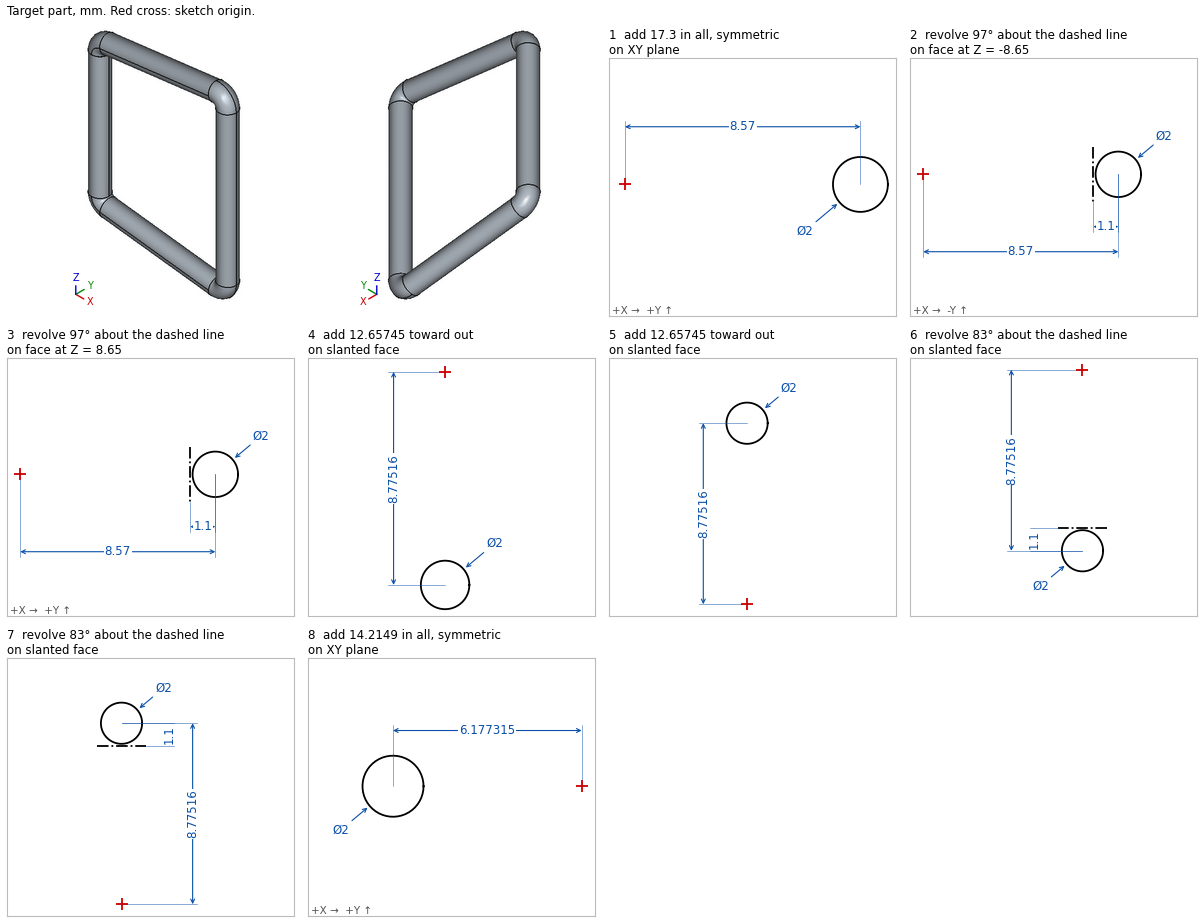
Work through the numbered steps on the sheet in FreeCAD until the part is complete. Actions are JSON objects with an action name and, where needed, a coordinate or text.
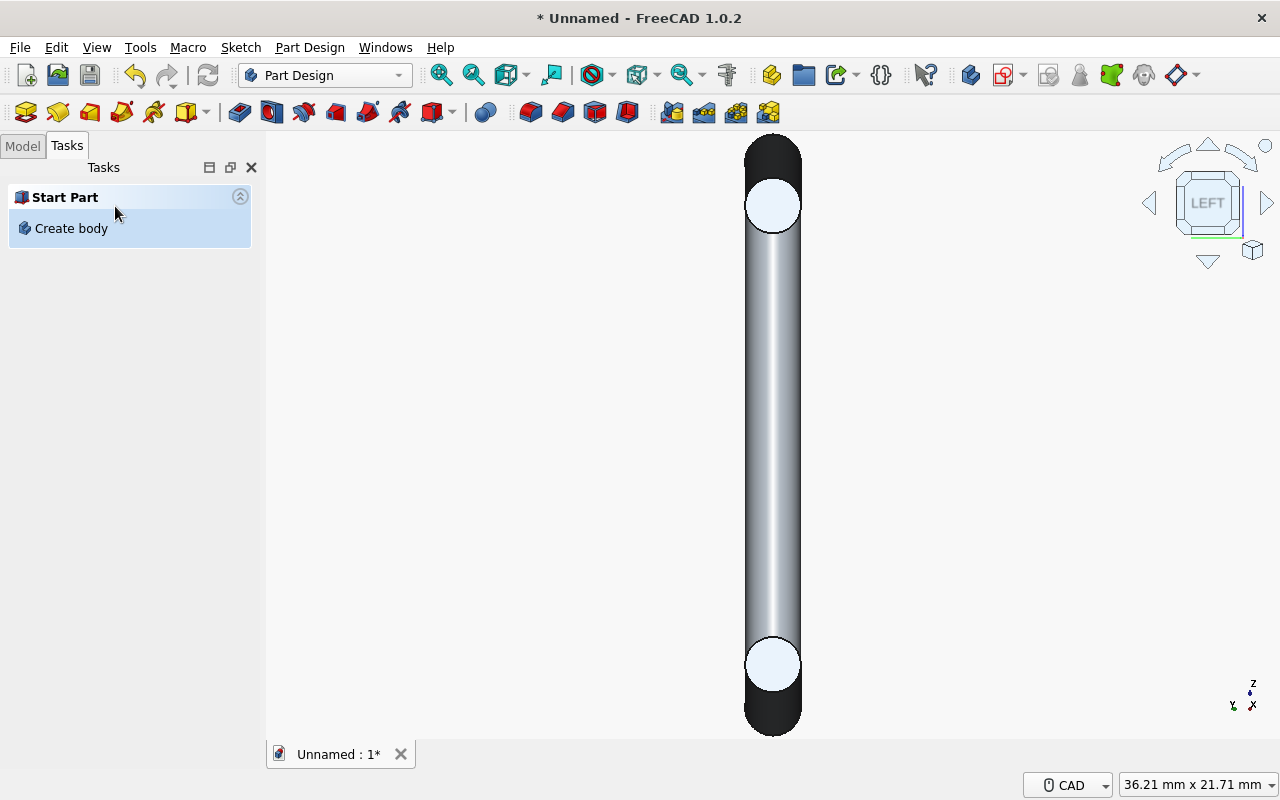
{"action": "left_click", "coordinate": [773, 664]}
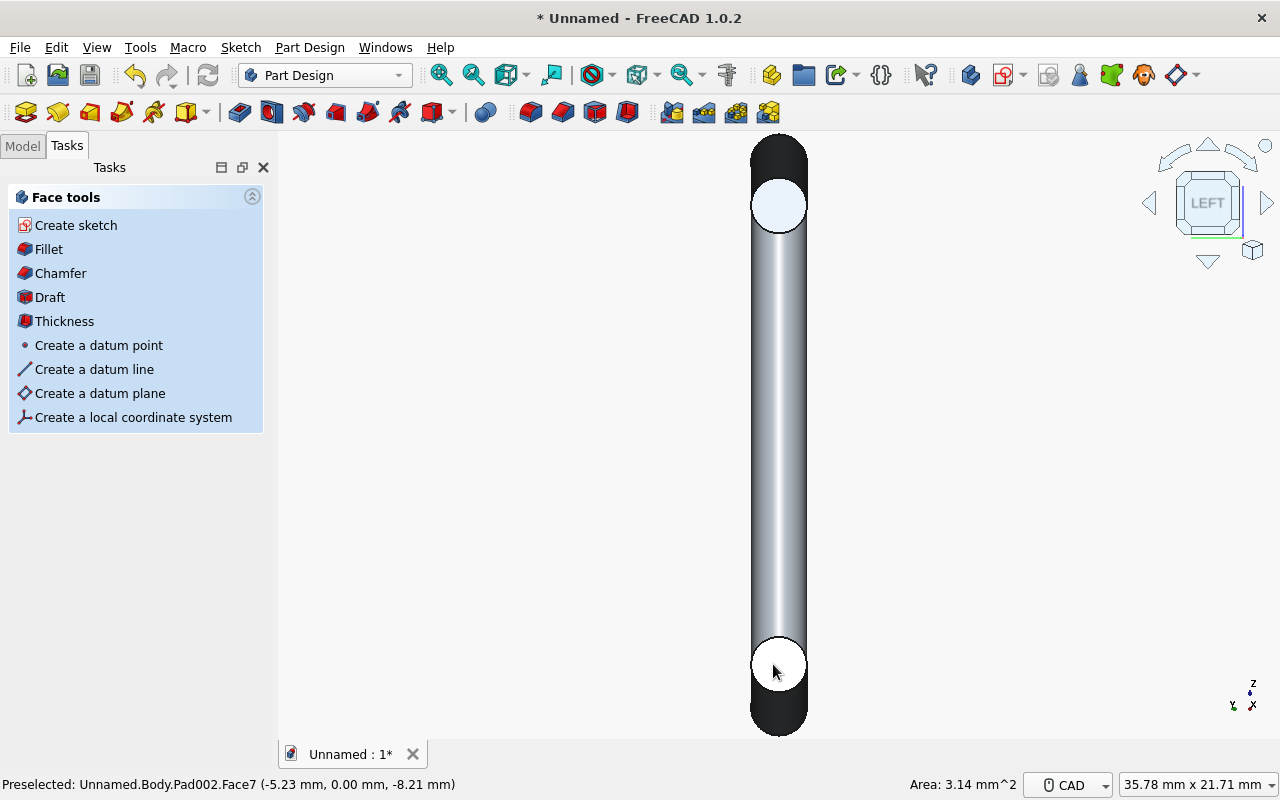
{"action": "left_click", "coordinate": [1004, 76]}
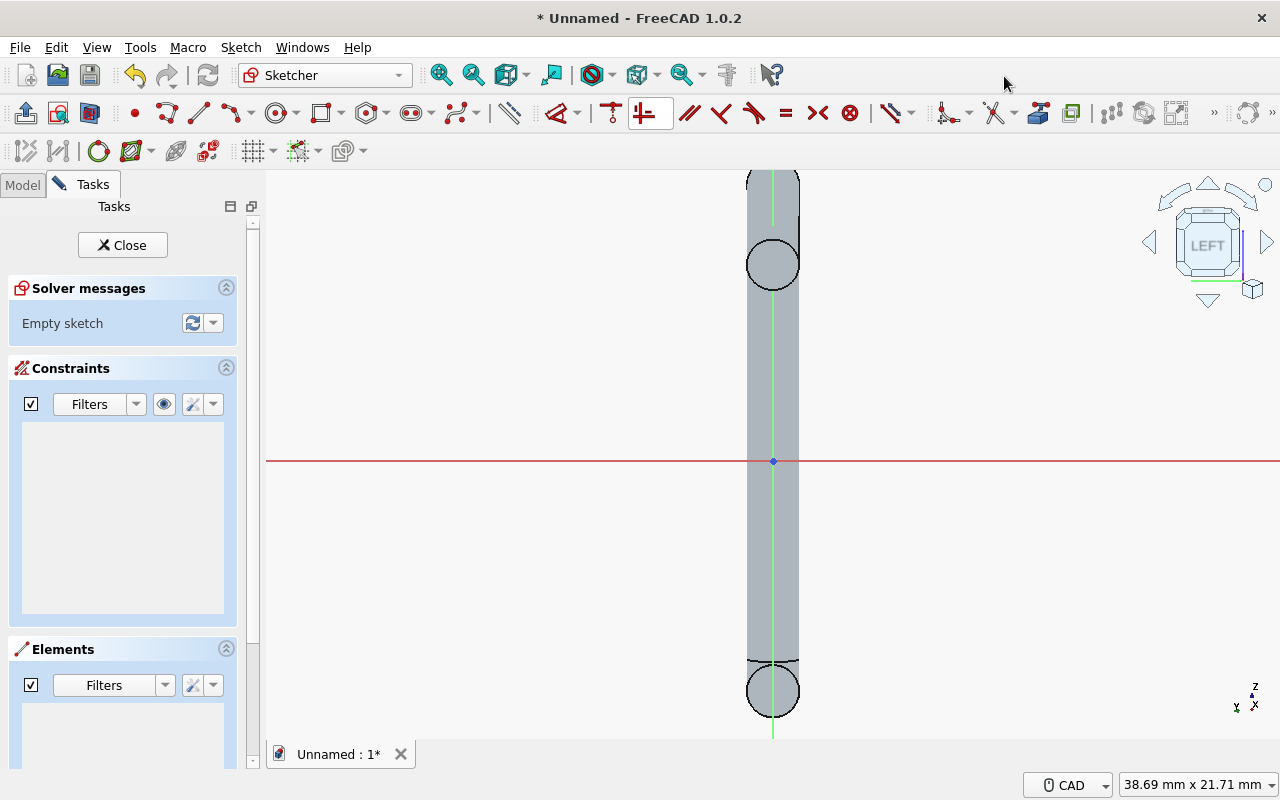
{"action": "scroll", "coordinate": [704, 454], "scroll_direction": "down", "scroll_amount": 5}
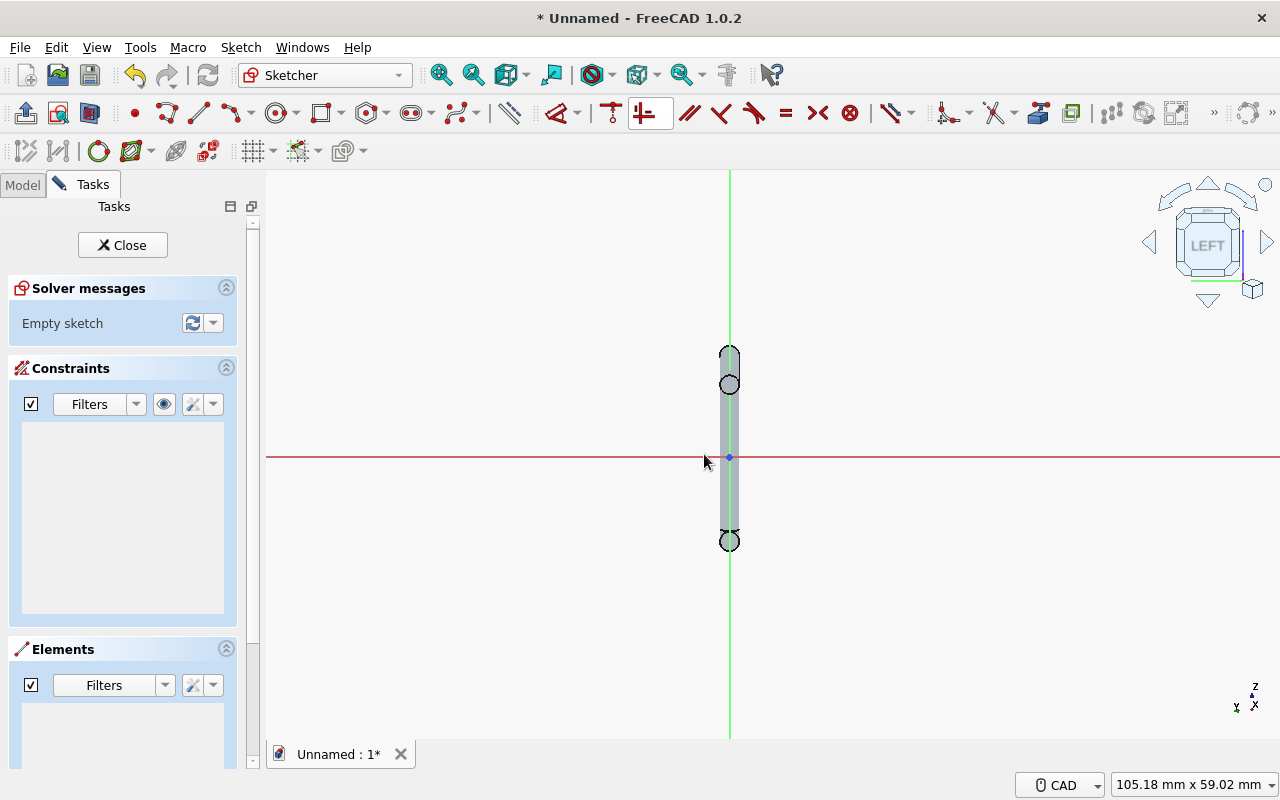
{"action": "scroll", "coordinate": [731, 547], "scroll_direction": "up", "scroll_amount": 14}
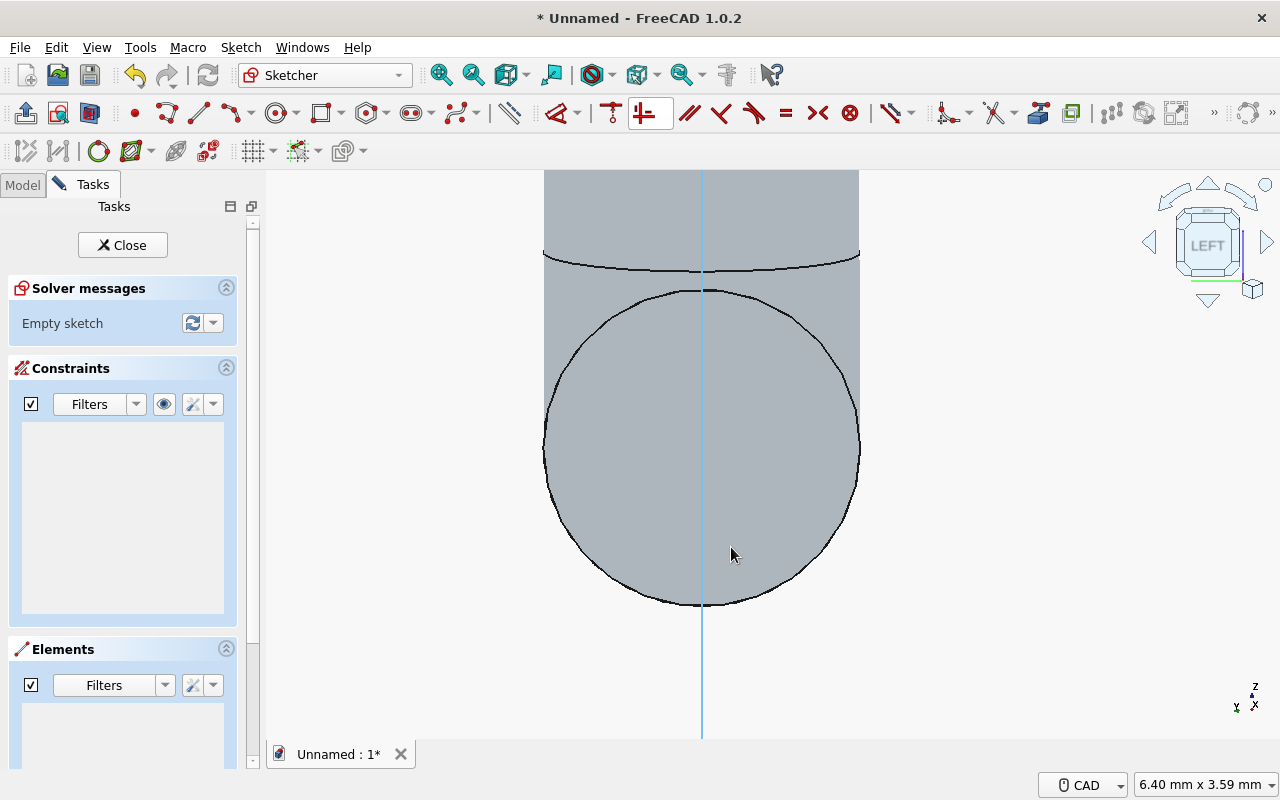
{"action": "left_click", "coordinate": [276, 114]}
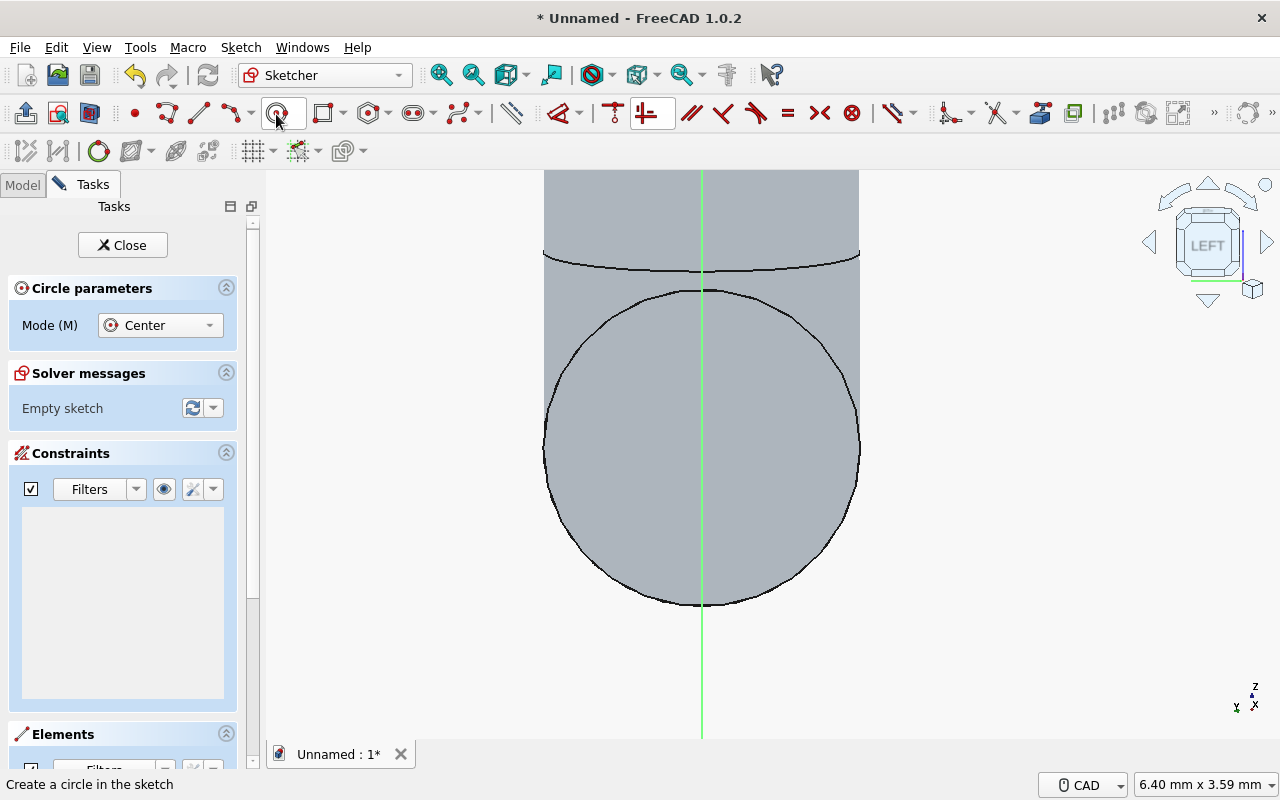
{"action": "left_click", "coordinate": [702, 448]}
{"action": "mouse_move", "coordinate": [814, 336]}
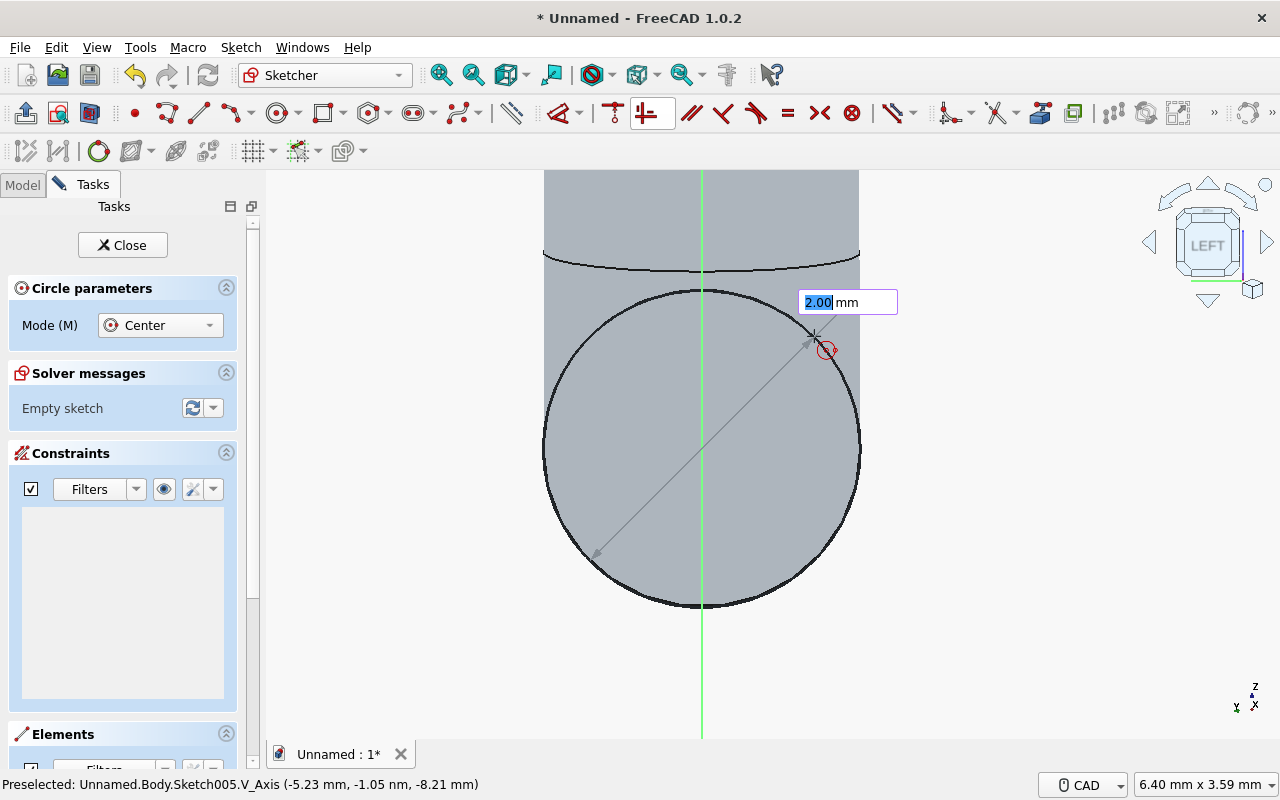
{"action": "type", "text": "2"}
{"action": "key", "text": "Return"}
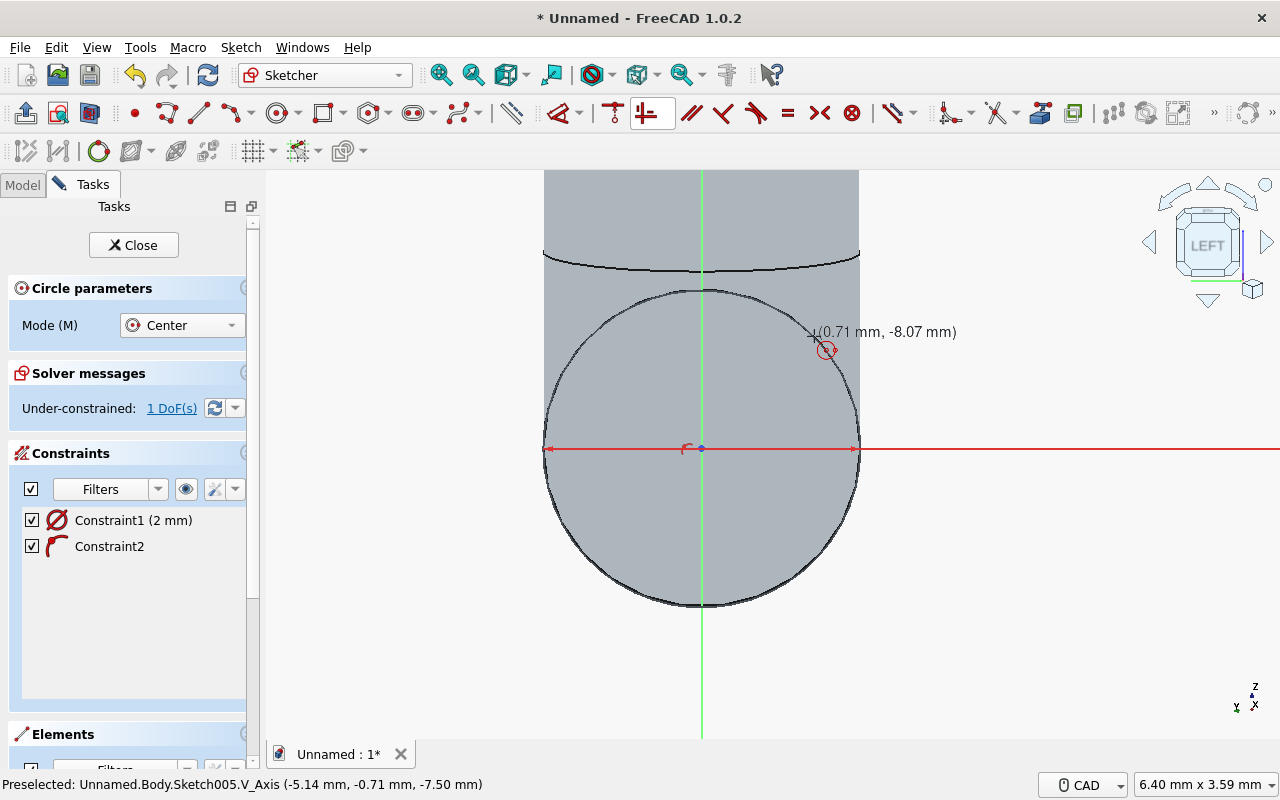
{"action": "left_click", "coordinate": [200, 114]}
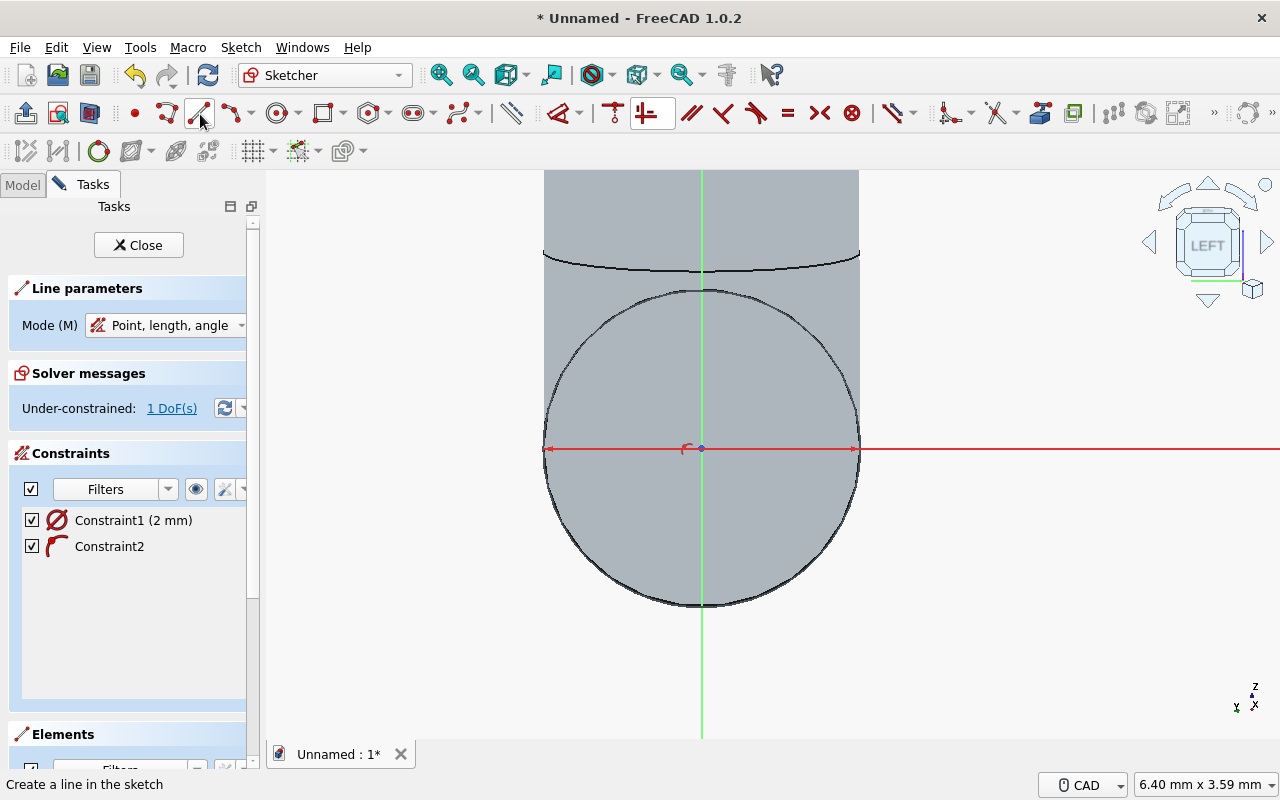
{"action": "left_click", "coordinate": [892, 274]}
{"action": "left_click", "coordinate": [512, 274]}
{"action": "key", "text": "Escape"}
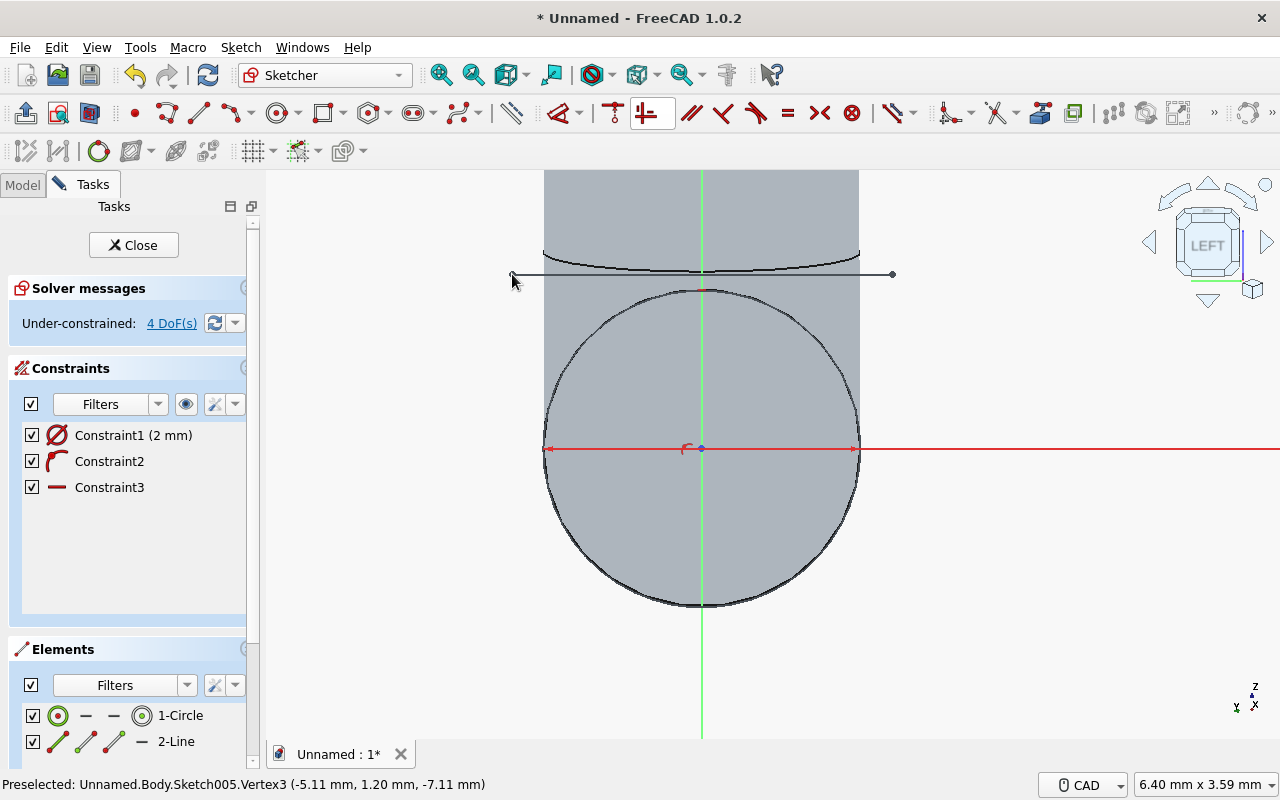
{"action": "left_click", "coordinate": [778, 275]}